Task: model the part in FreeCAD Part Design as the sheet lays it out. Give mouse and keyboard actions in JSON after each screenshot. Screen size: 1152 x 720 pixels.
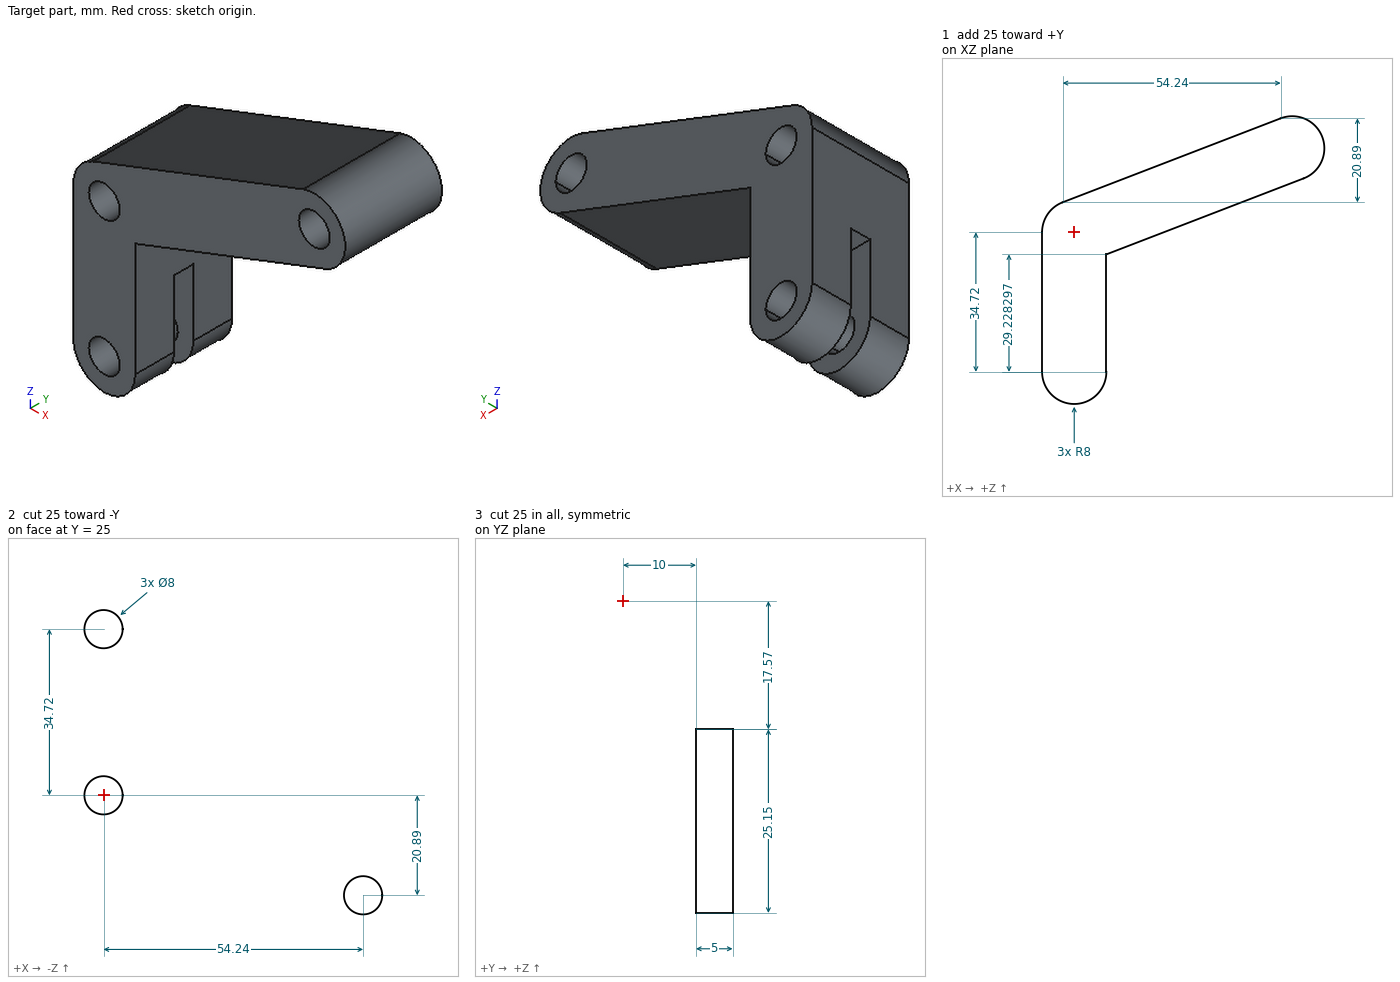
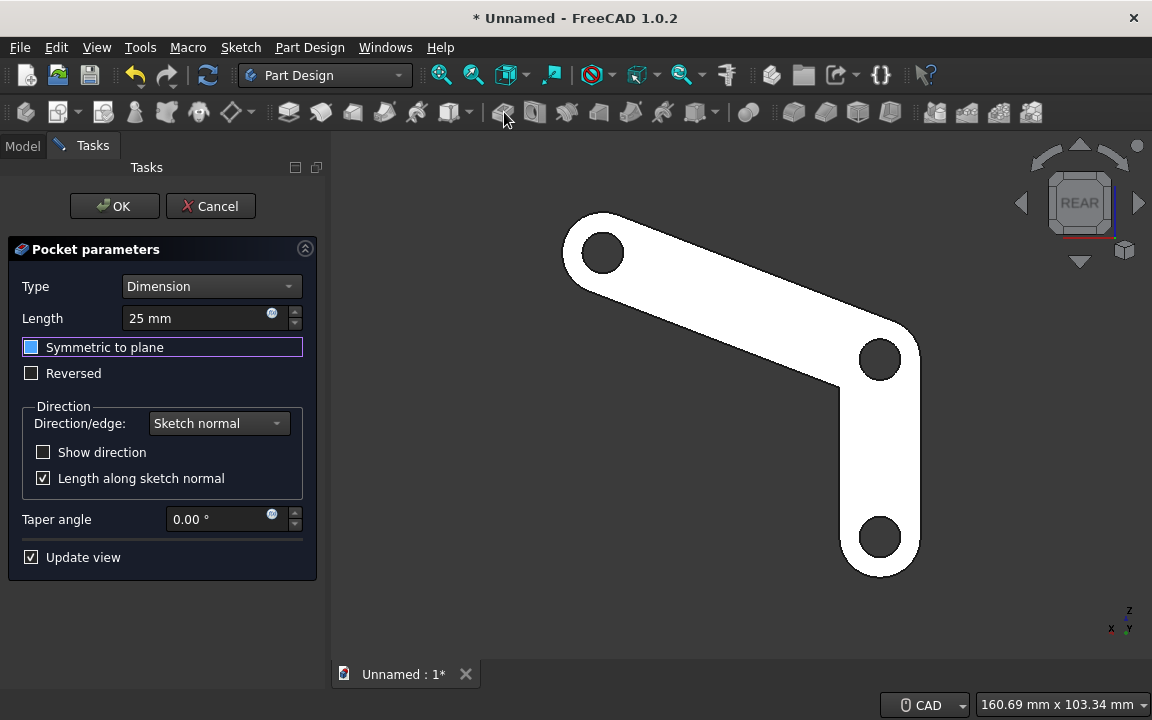
{"action": "left_click", "coordinate": [115, 206]}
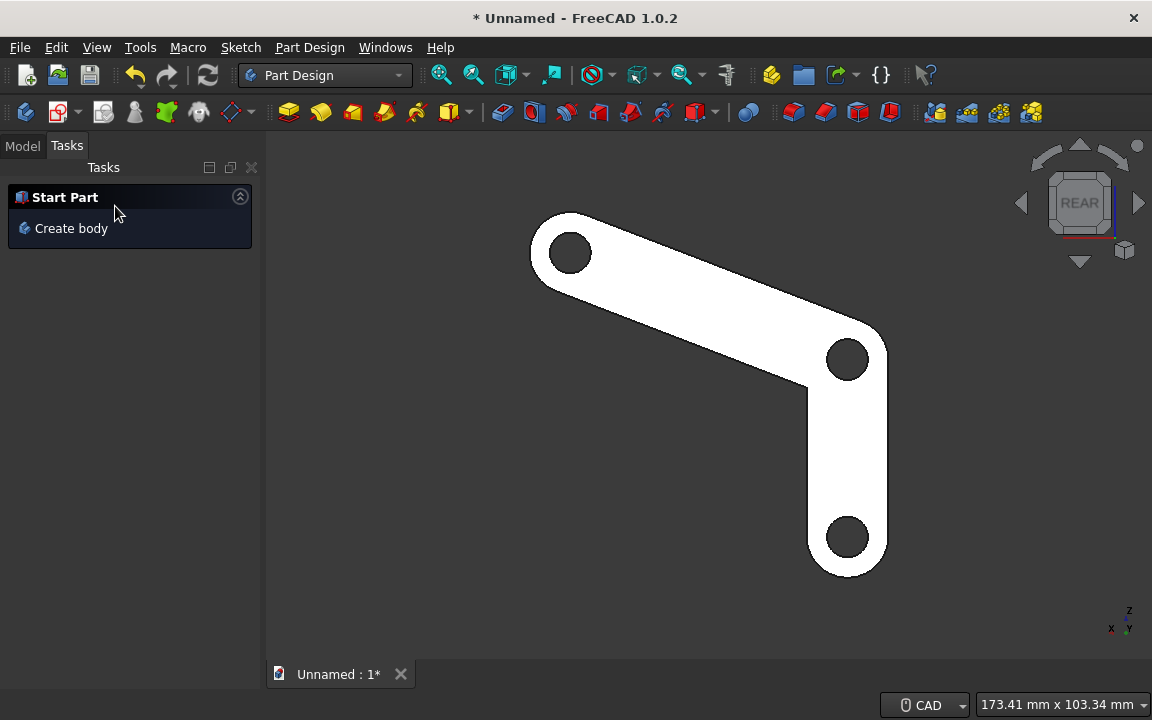
{"action": "left_click", "coordinate": [58, 112]}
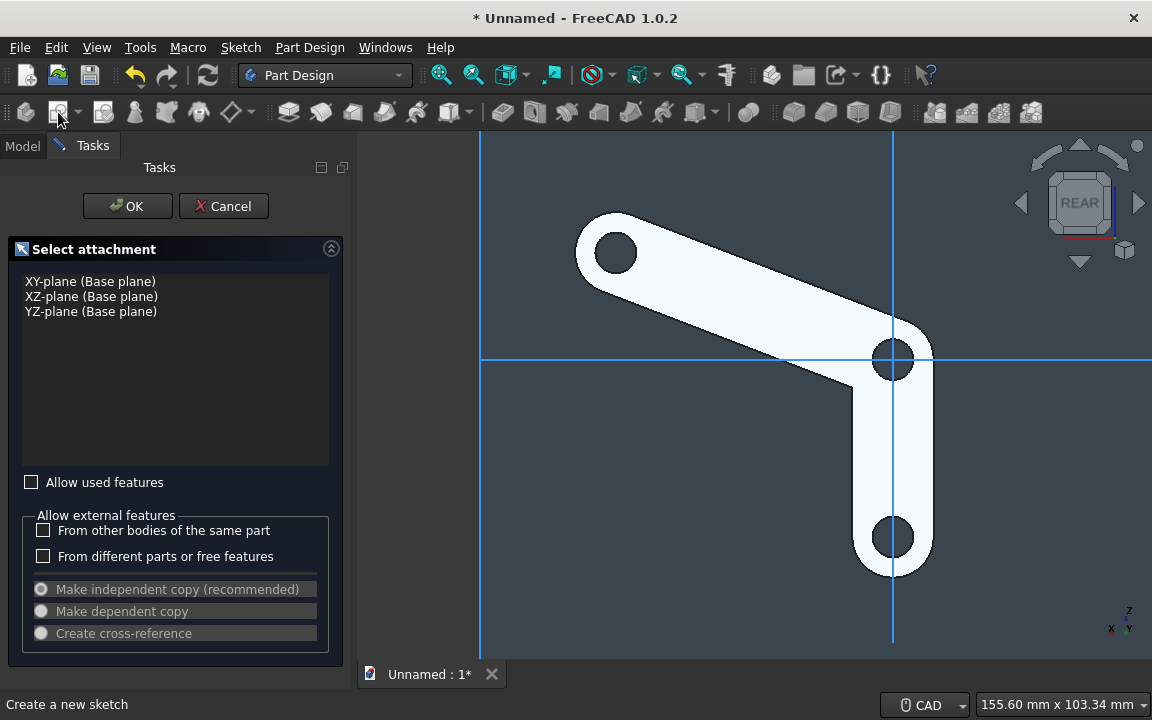
{"action": "left_click", "coordinate": [82, 312]}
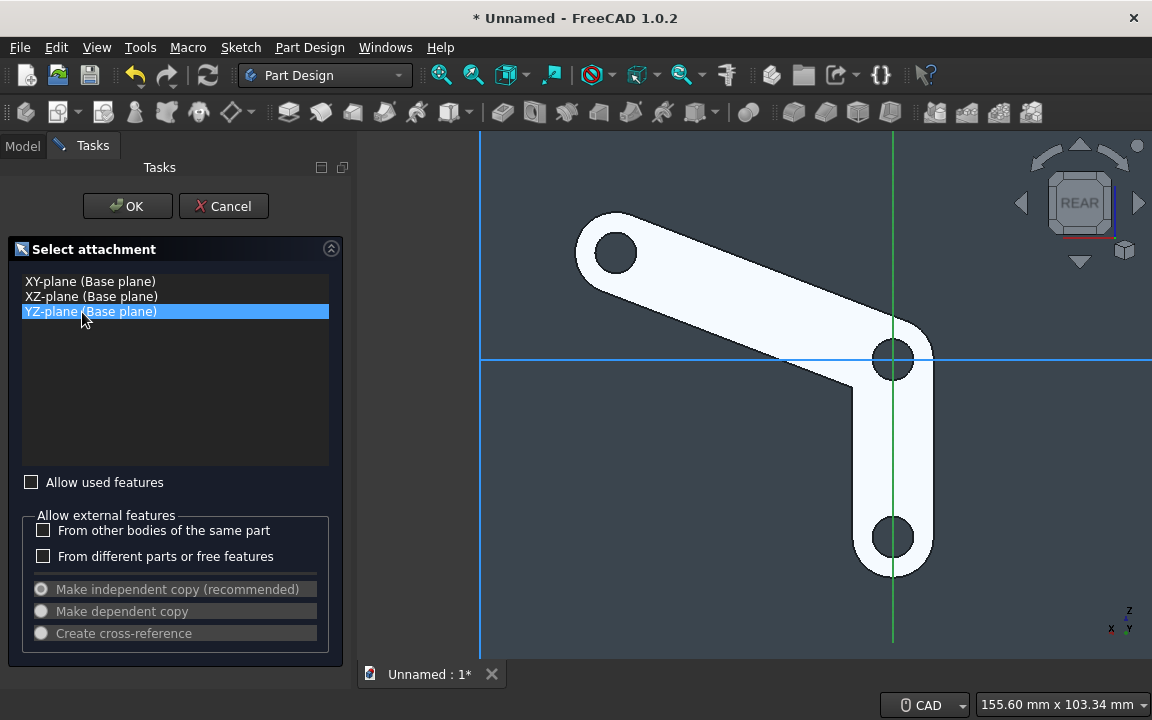
{"action": "left_click", "coordinate": [128, 206]}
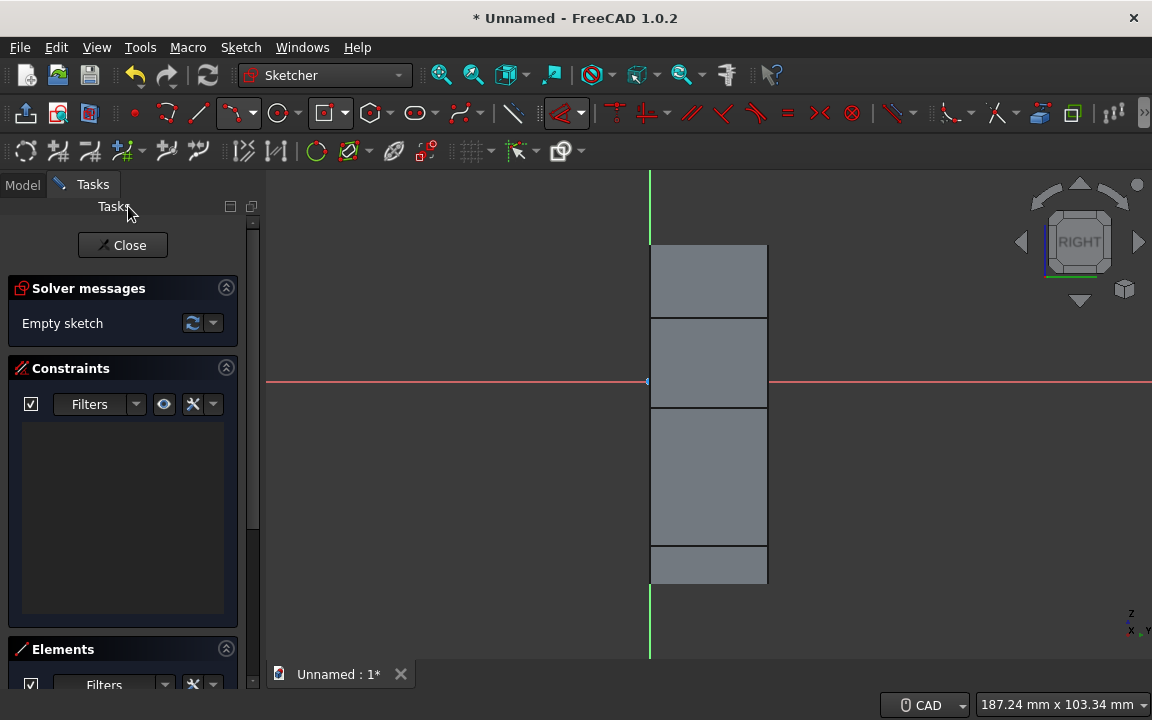
{"action": "left_click", "coordinate": [90, 114]}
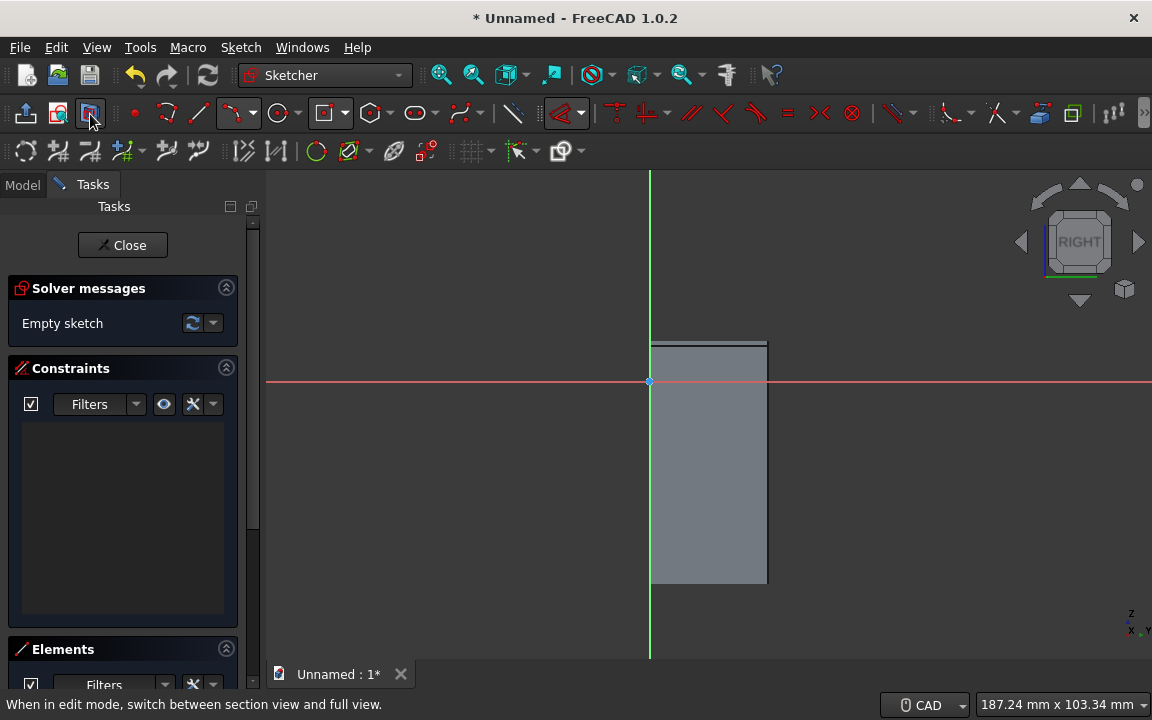
{"action": "scroll", "coordinate": [777, 622], "scroll_direction": "up", "scroll_amount": 2}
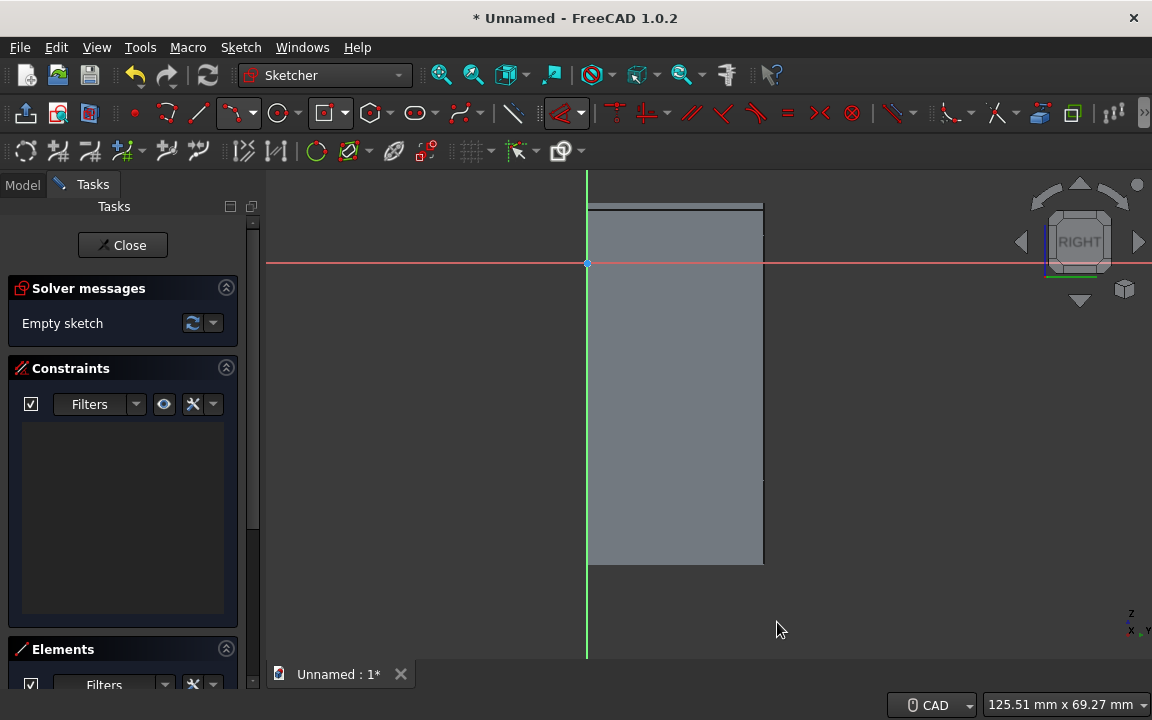
{"action": "key", "text": "g r"}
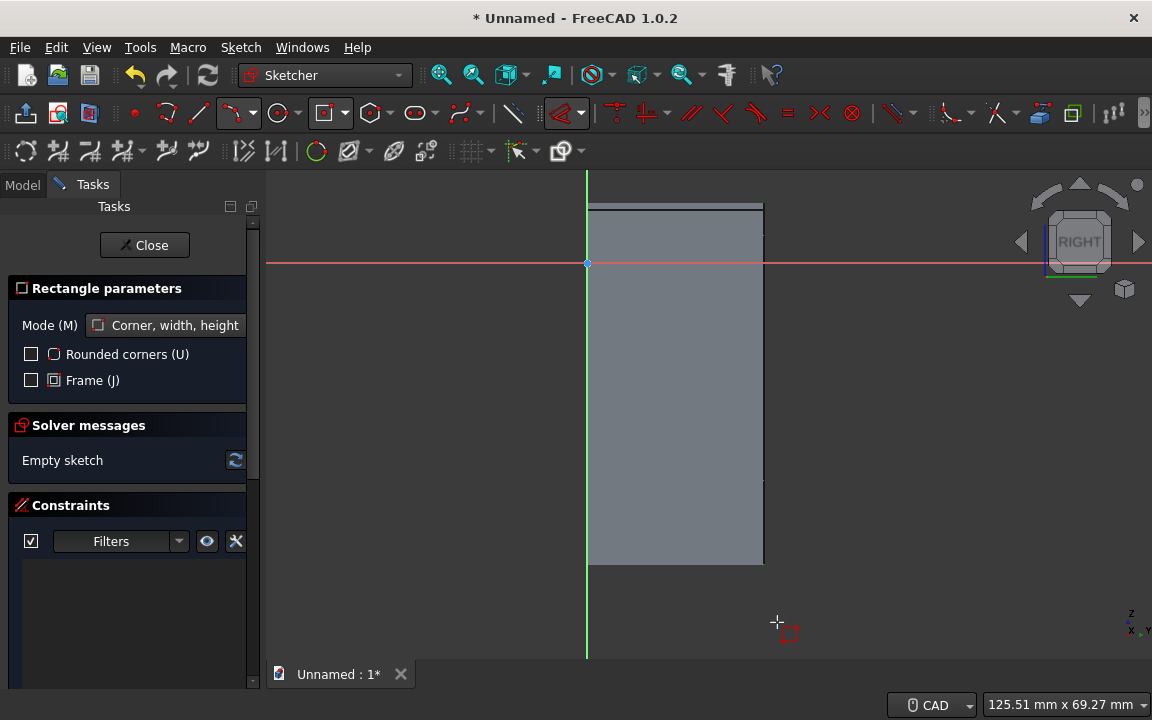
{"action": "left_click", "coordinate": [658, 387]}
{"action": "left_click", "coordinate": [693, 565]}
{"action": "key", "text": "Escape"}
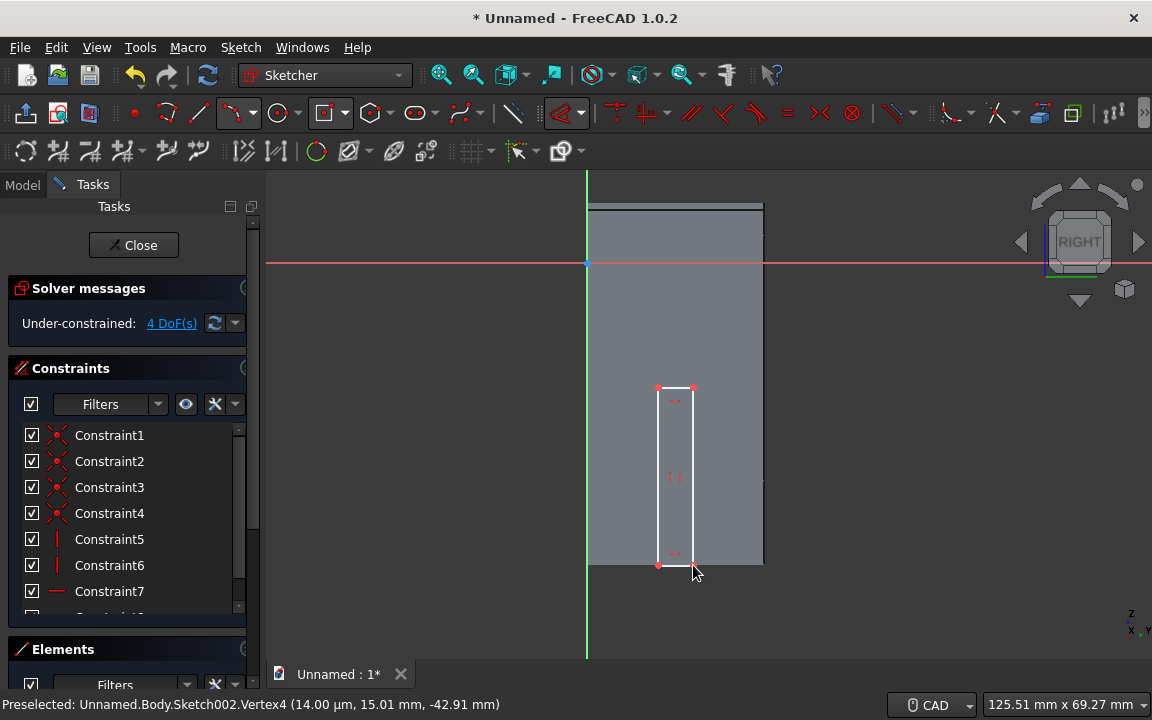
{"action": "scroll", "coordinate": [669, 566], "scroll_direction": "up", "scroll_amount": 2}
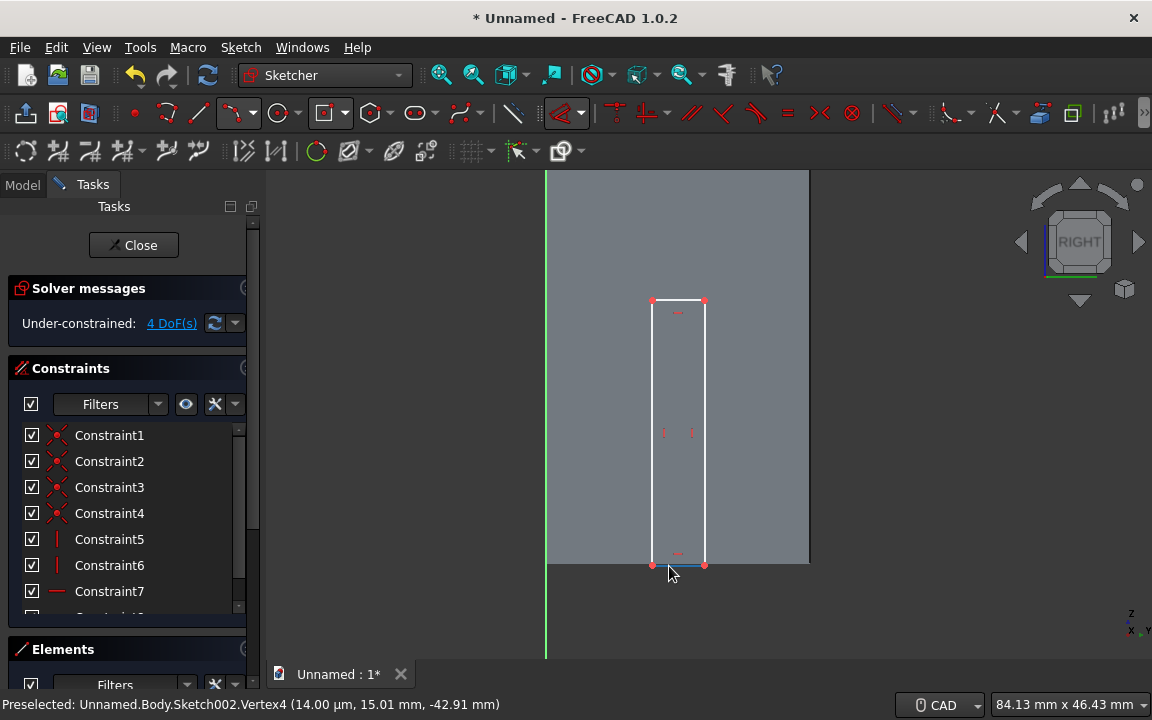
{"action": "left_click", "coordinate": [668, 566]}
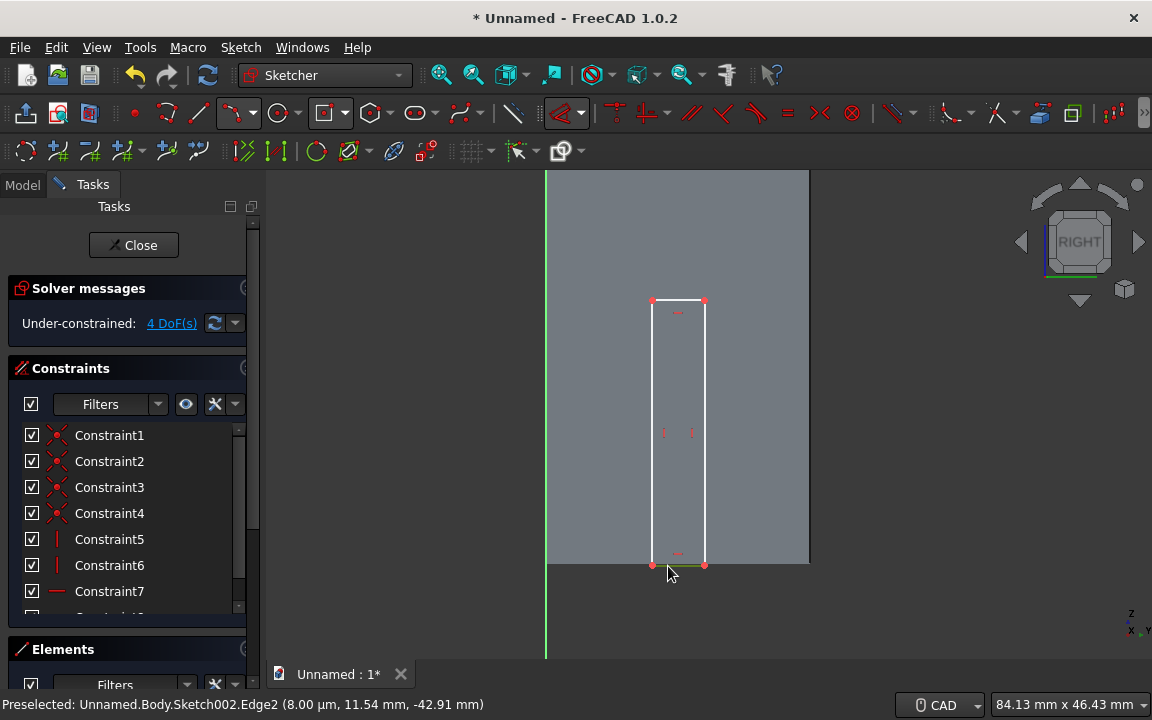
{"action": "left_click", "coordinate": [584, 114]}